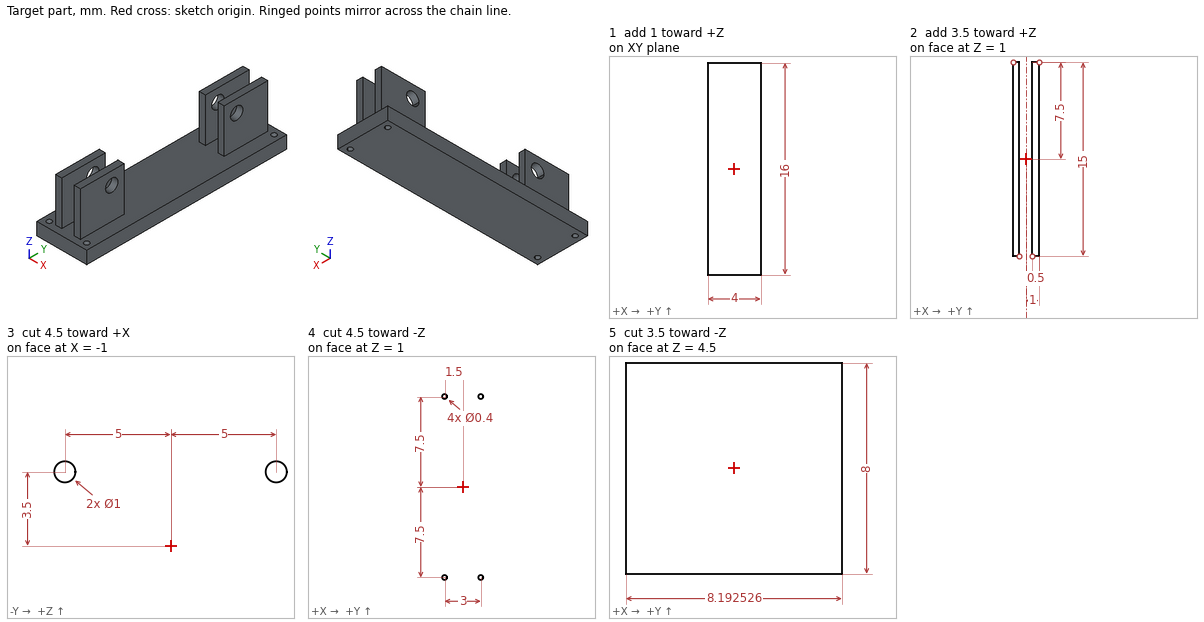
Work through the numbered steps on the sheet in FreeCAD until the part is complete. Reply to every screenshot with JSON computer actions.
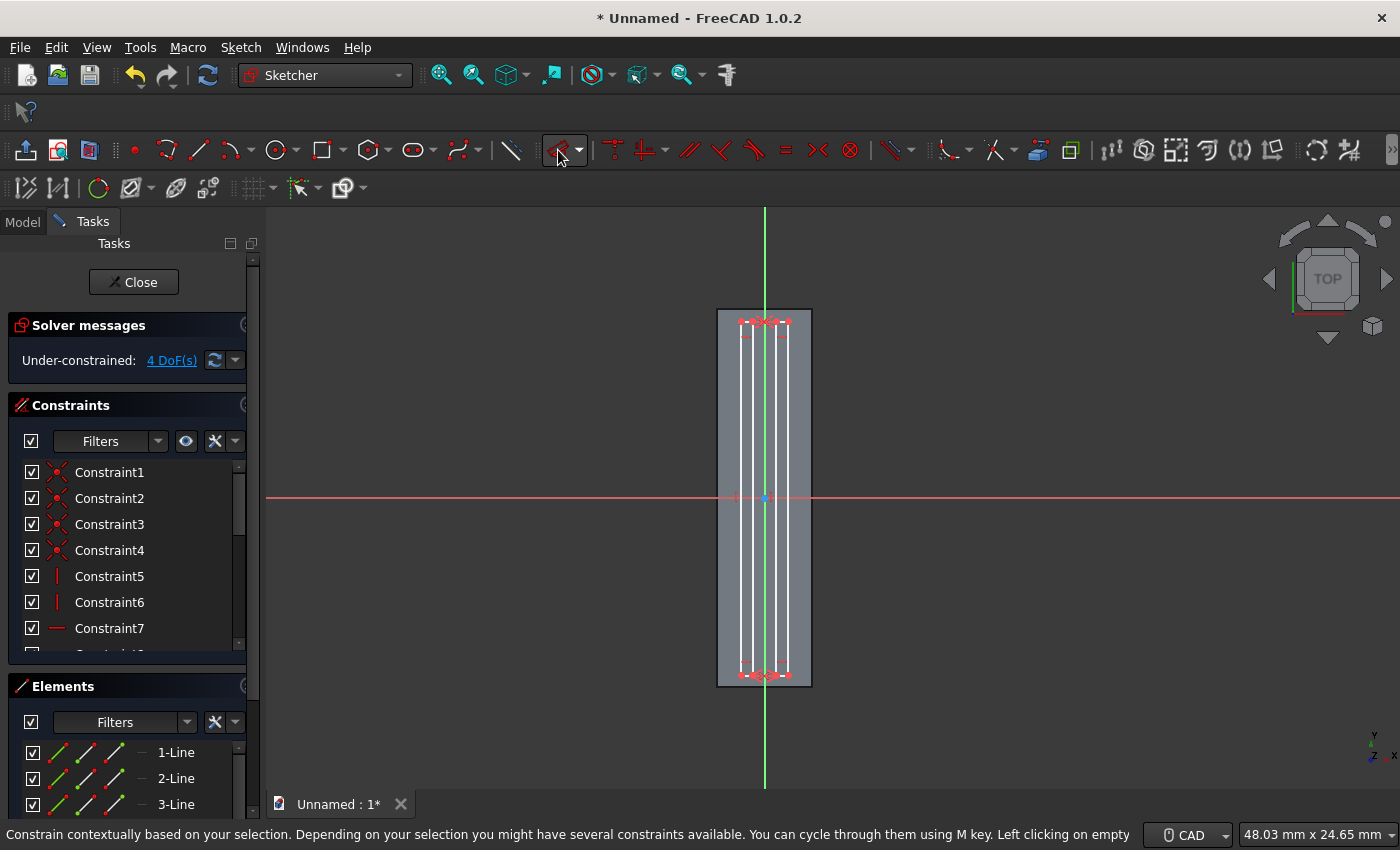
{"action": "left_click", "coordinate": [776, 428]}
{"action": "left_click", "coordinate": [810, 417]}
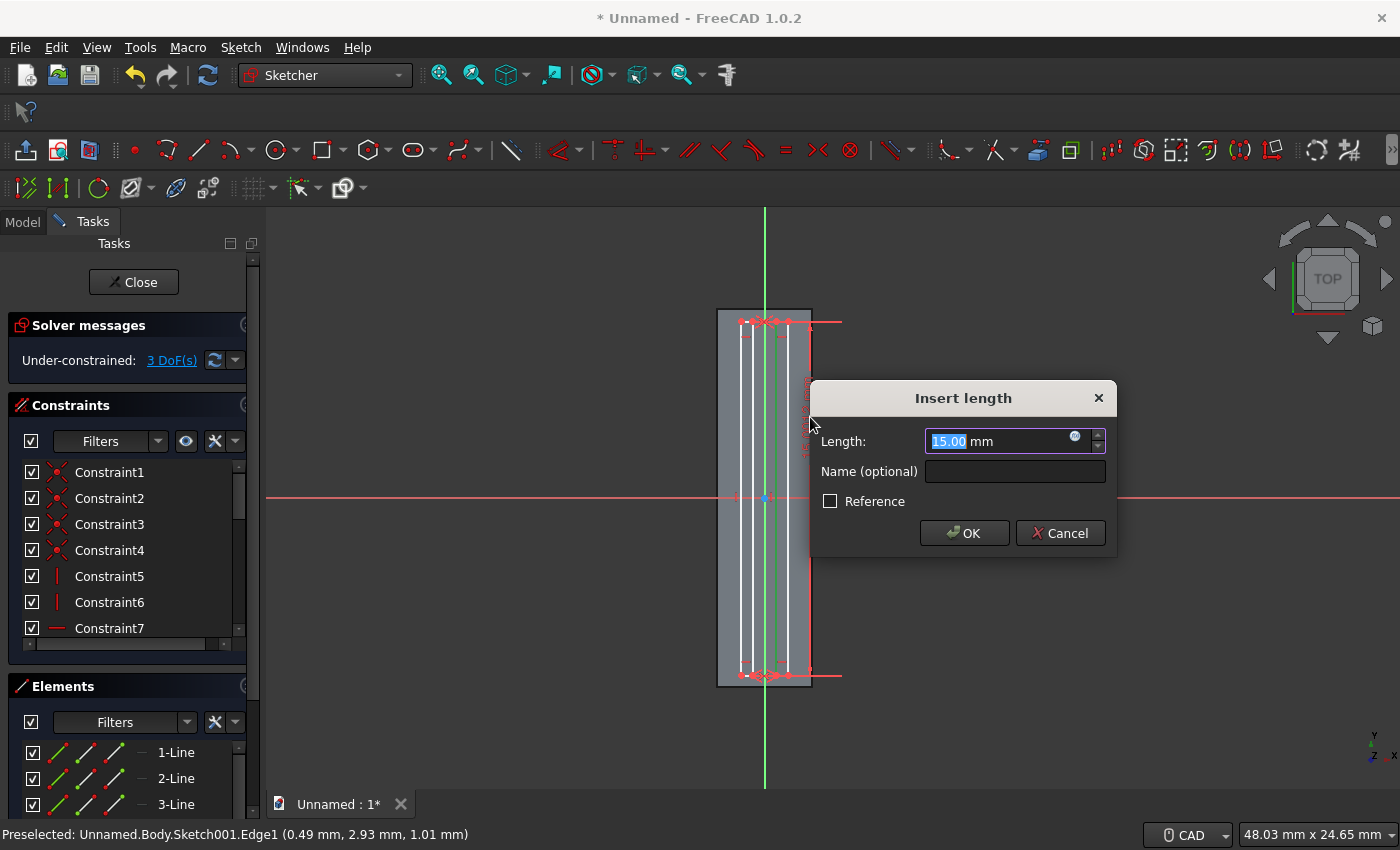
{"action": "type", "text": "15"}
{"action": "key", "text": "Return"}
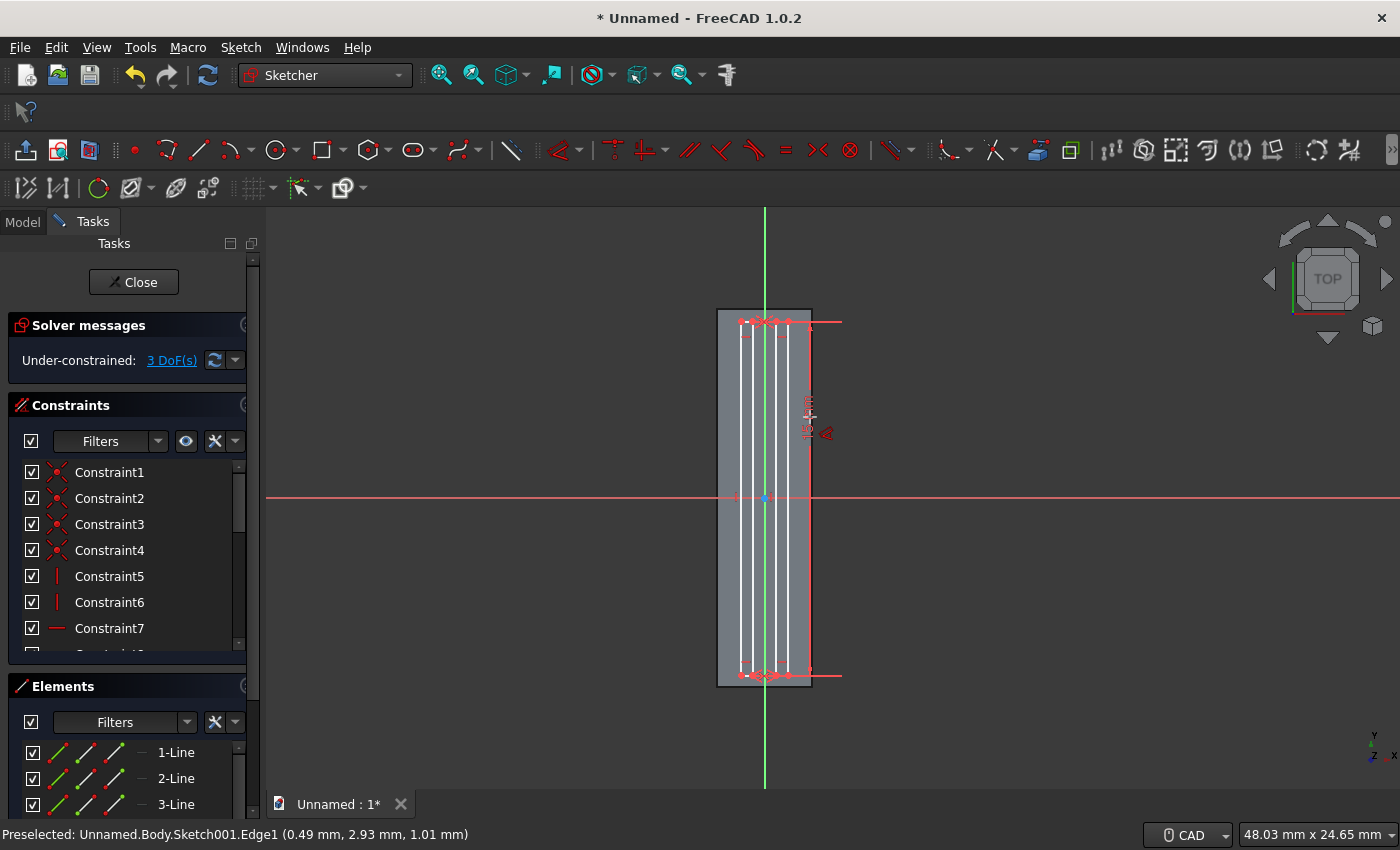
{"action": "scroll", "coordinate": [788, 676], "scroll_direction": "up", "scroll_amount": 3}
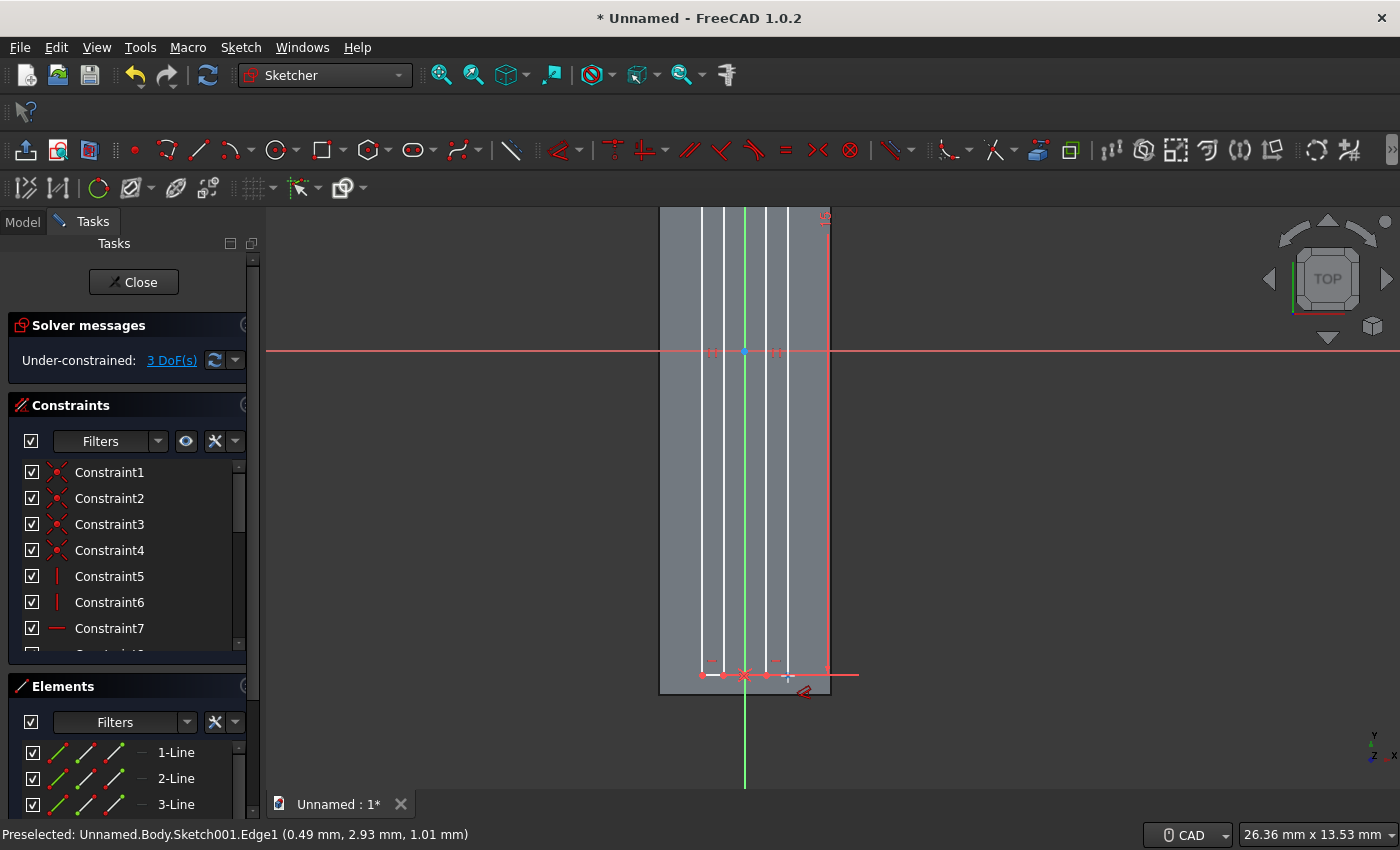
{"action": "left_click", "coordinate": [788, 675]}
{"action": "left_click", "coordinate": [766, 709]}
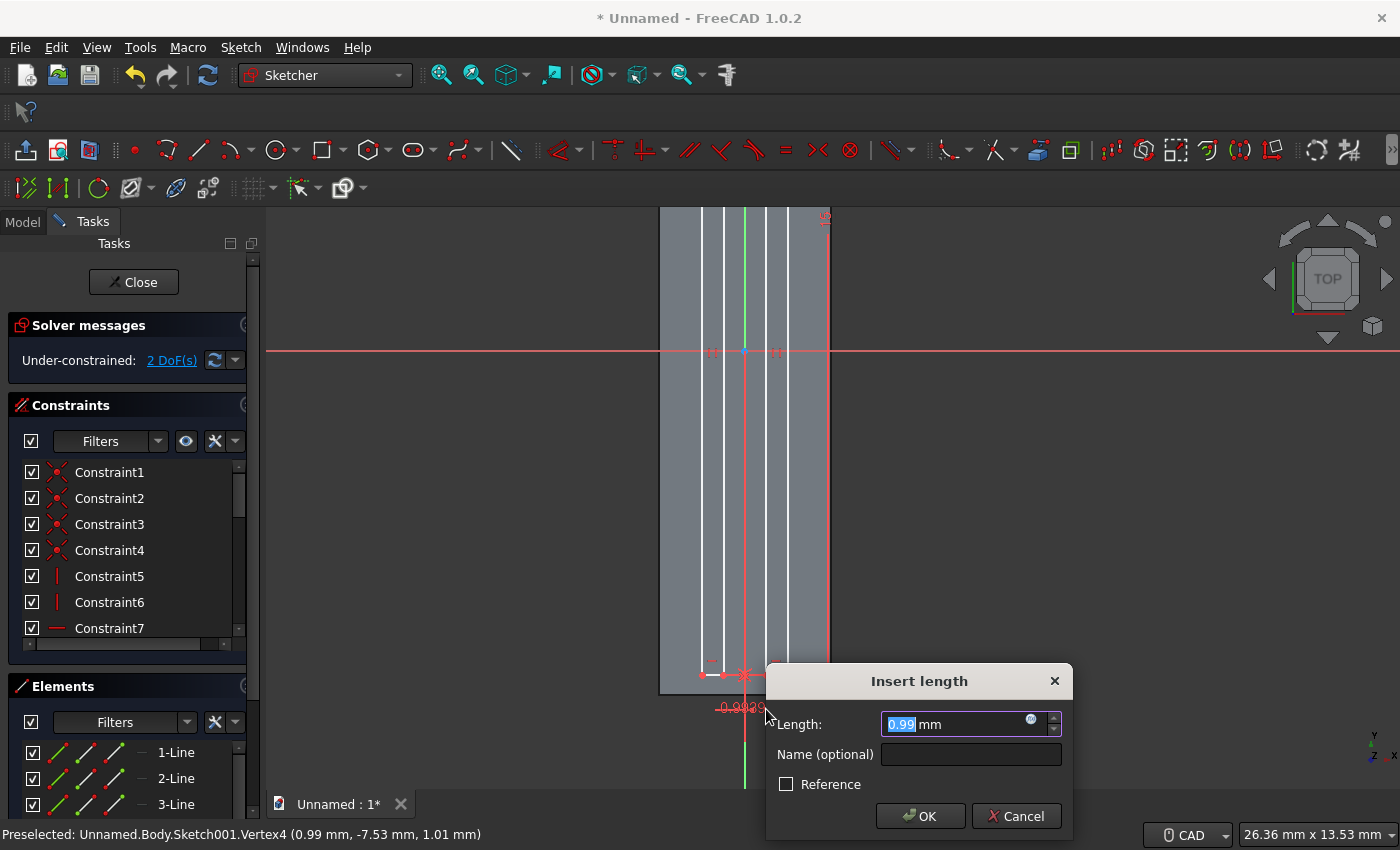
{"action": "type", "text": "1"}
{"action": "key", "text": "Return"}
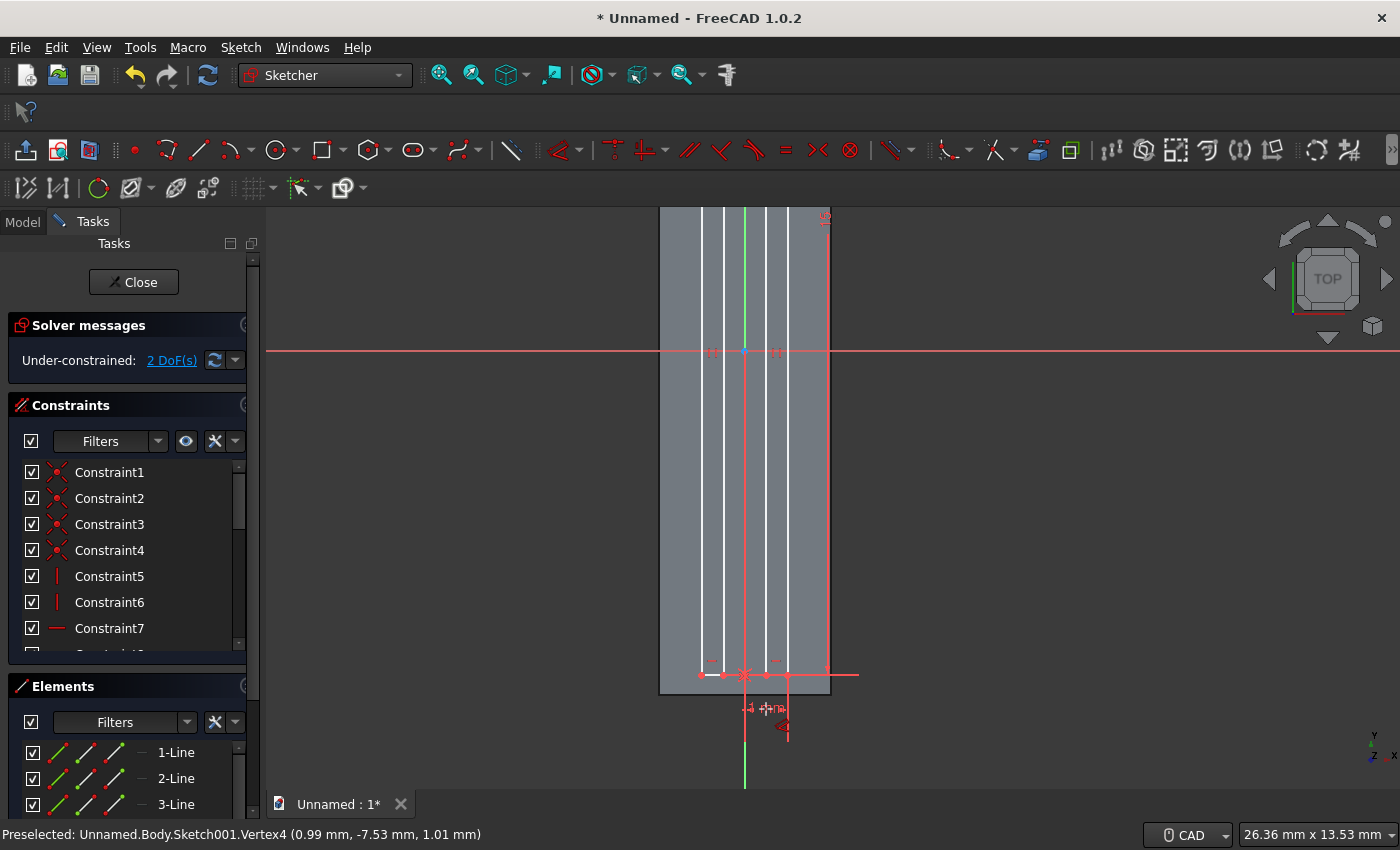
{"action": "scroll", "coordinate": [777, 675], "scroll_direction": "up", "scroll_amount": 4}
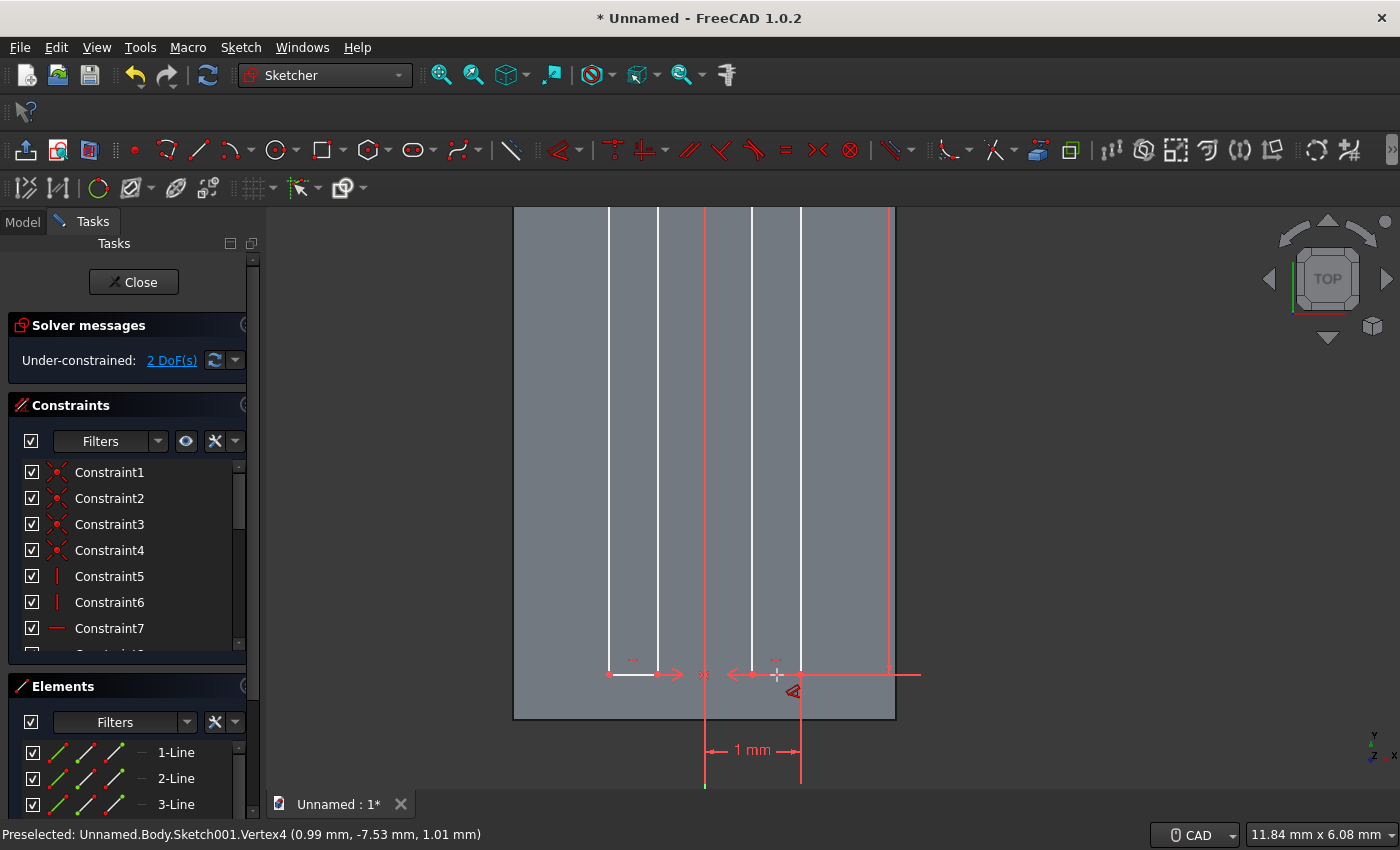
{"action": "left_click", "coordinate": [776, 675]}
{"action": "left_click", "coordinate": [776, 709]}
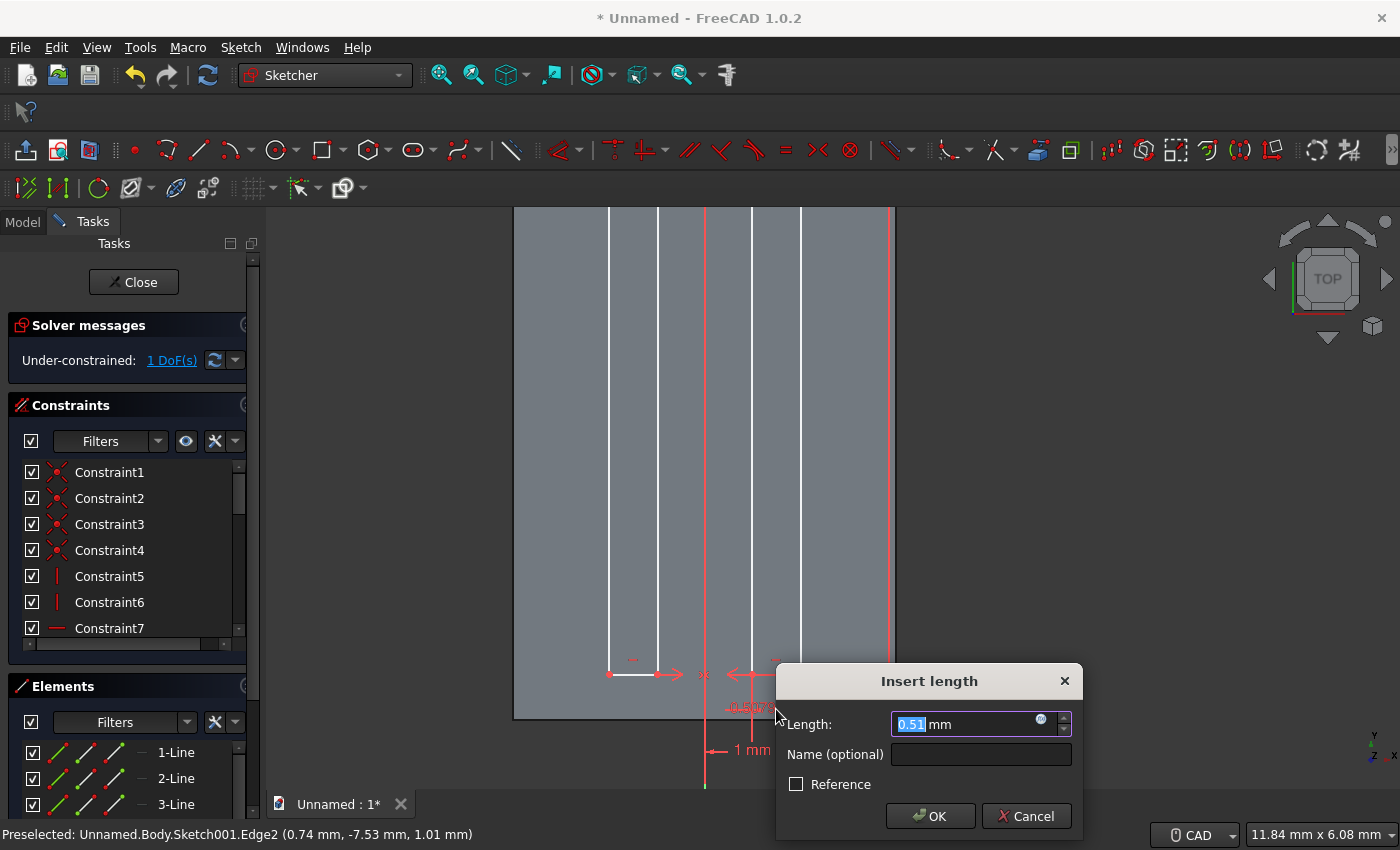
{"action": "type", "text": "0.5"}
{"action": "key", "text": "Return"}